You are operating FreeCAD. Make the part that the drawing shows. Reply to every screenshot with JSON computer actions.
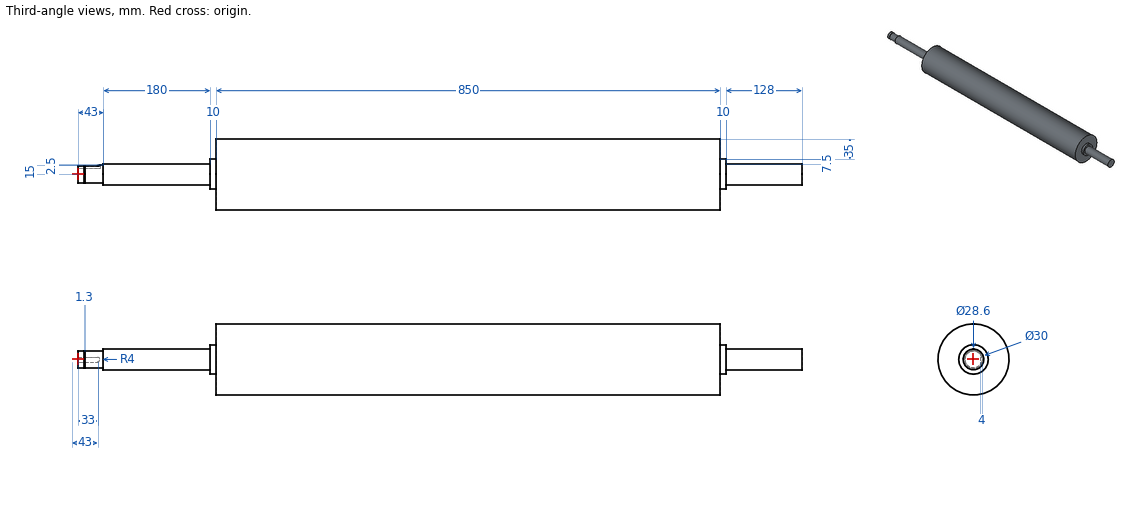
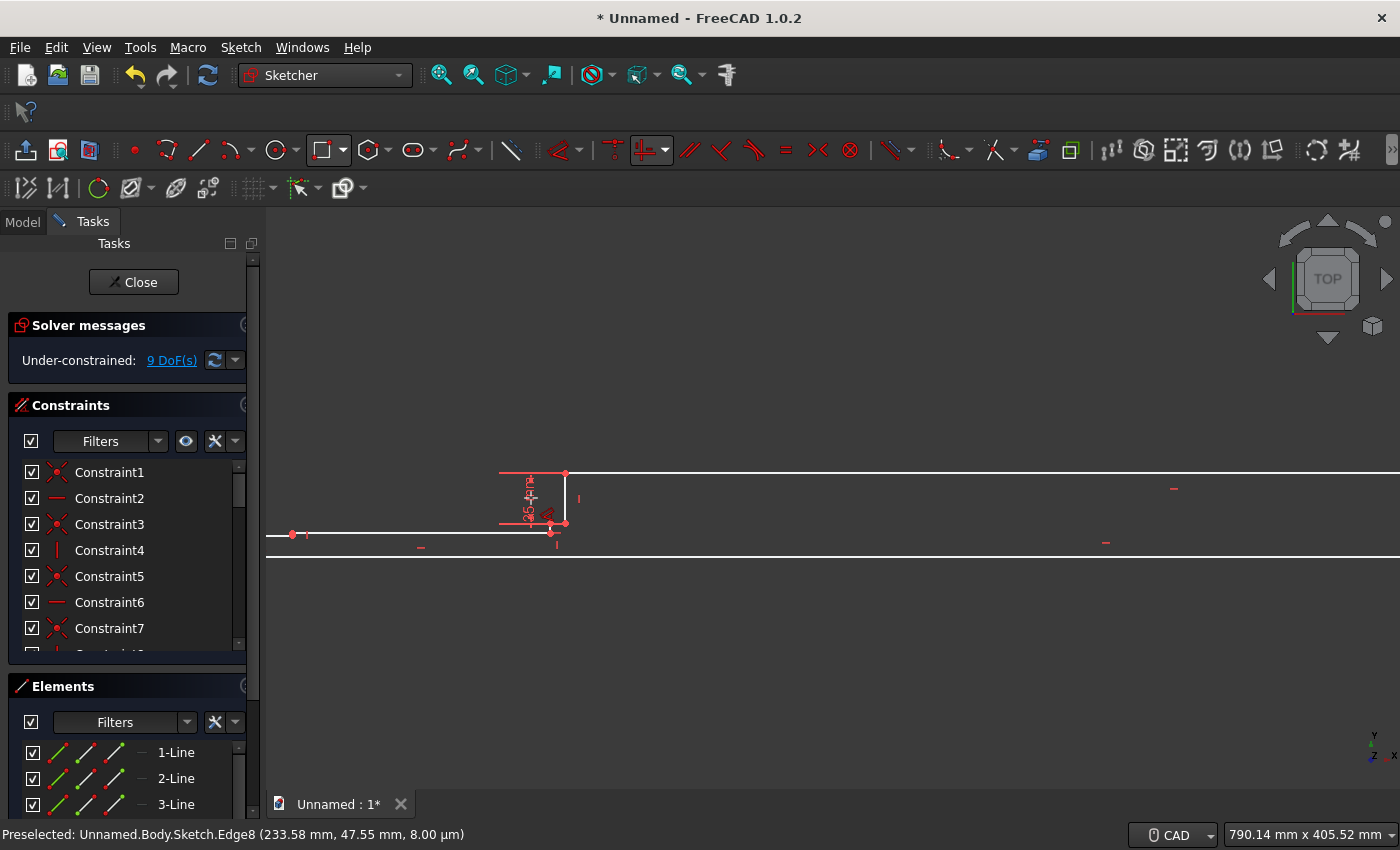
{"action": "scroll", "coordinate": [558, 524], "scroll_direction": "up", "scroll_amount": 6}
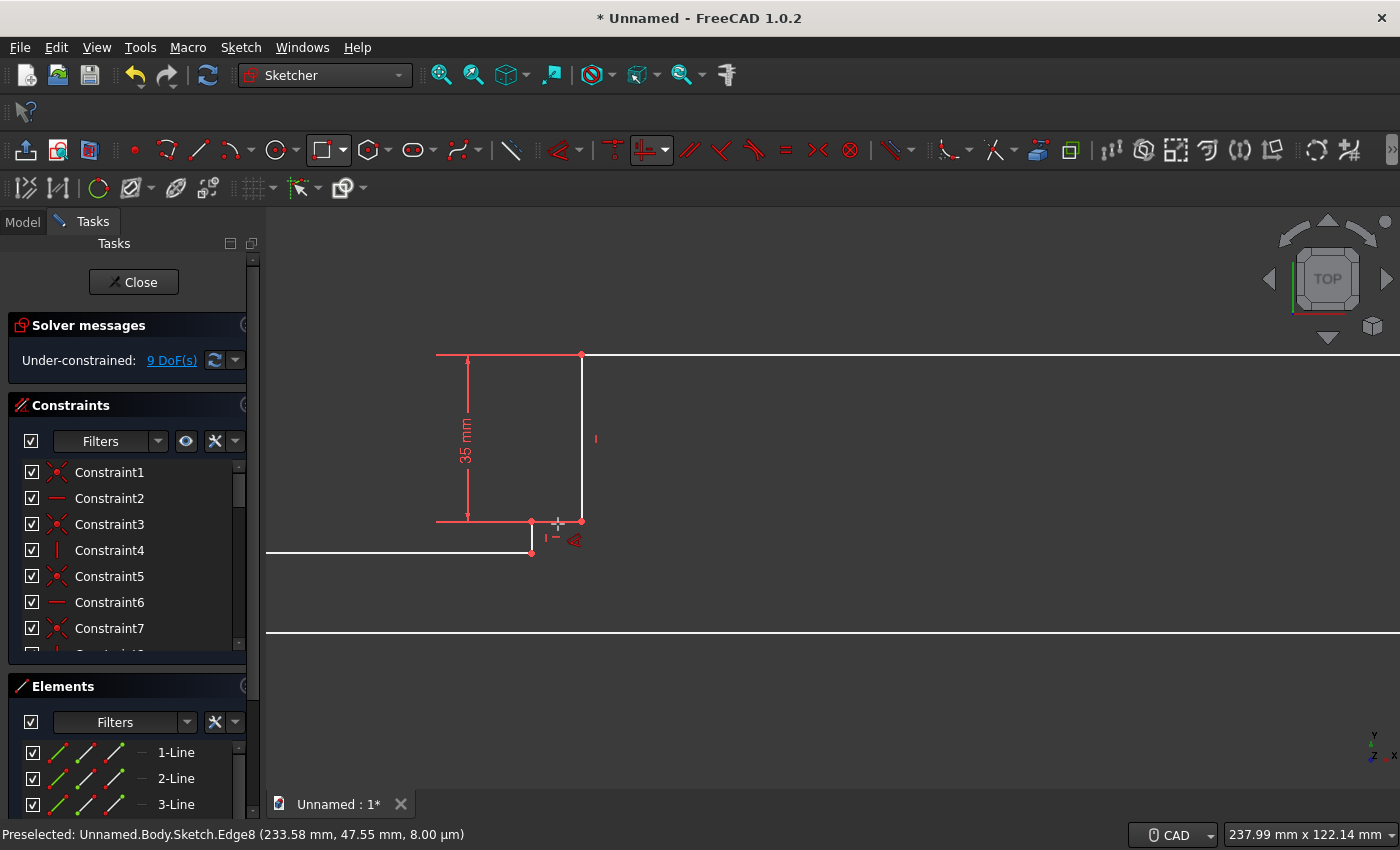
{"action": "left_click", "coordinate": [557, 522]}
{"action": "left_click", "coordinate": [557, 556]}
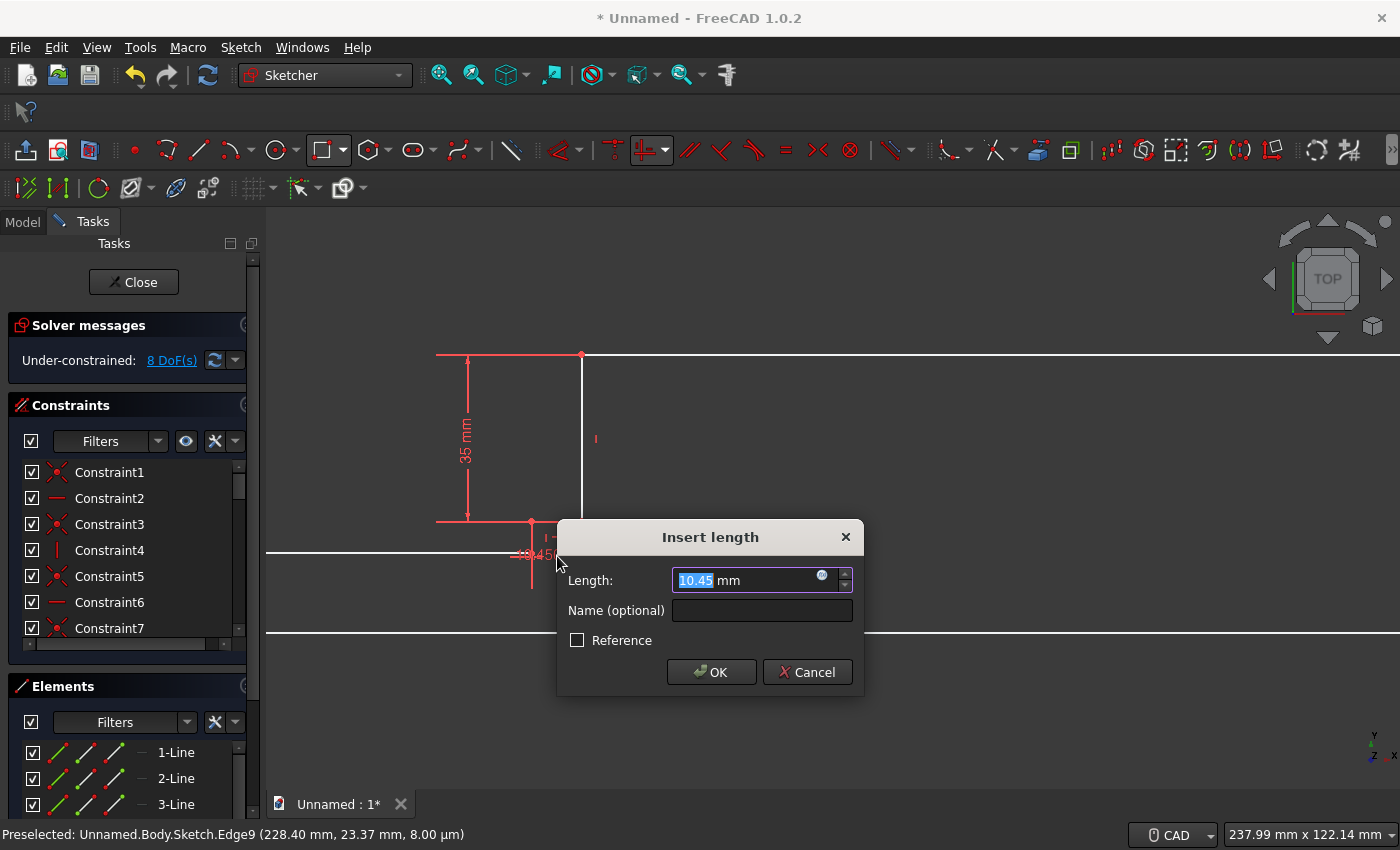
{"action": "type", "text": "10"}
{"action": "key", "text": "Return"}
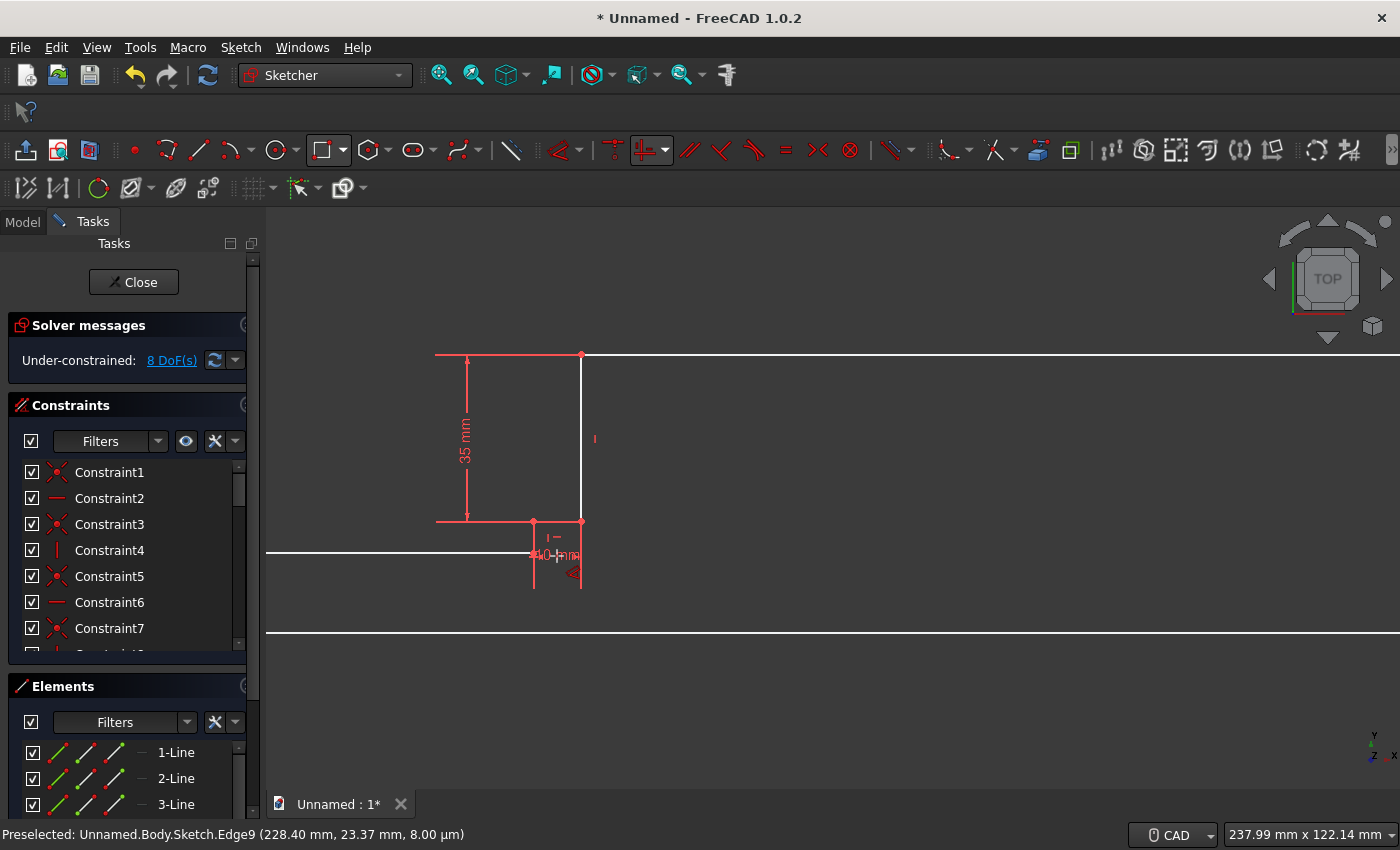
{"action": "scroll", "coordinate": [563, 499], "scroll_direction": "down", "scroll_amount": 11}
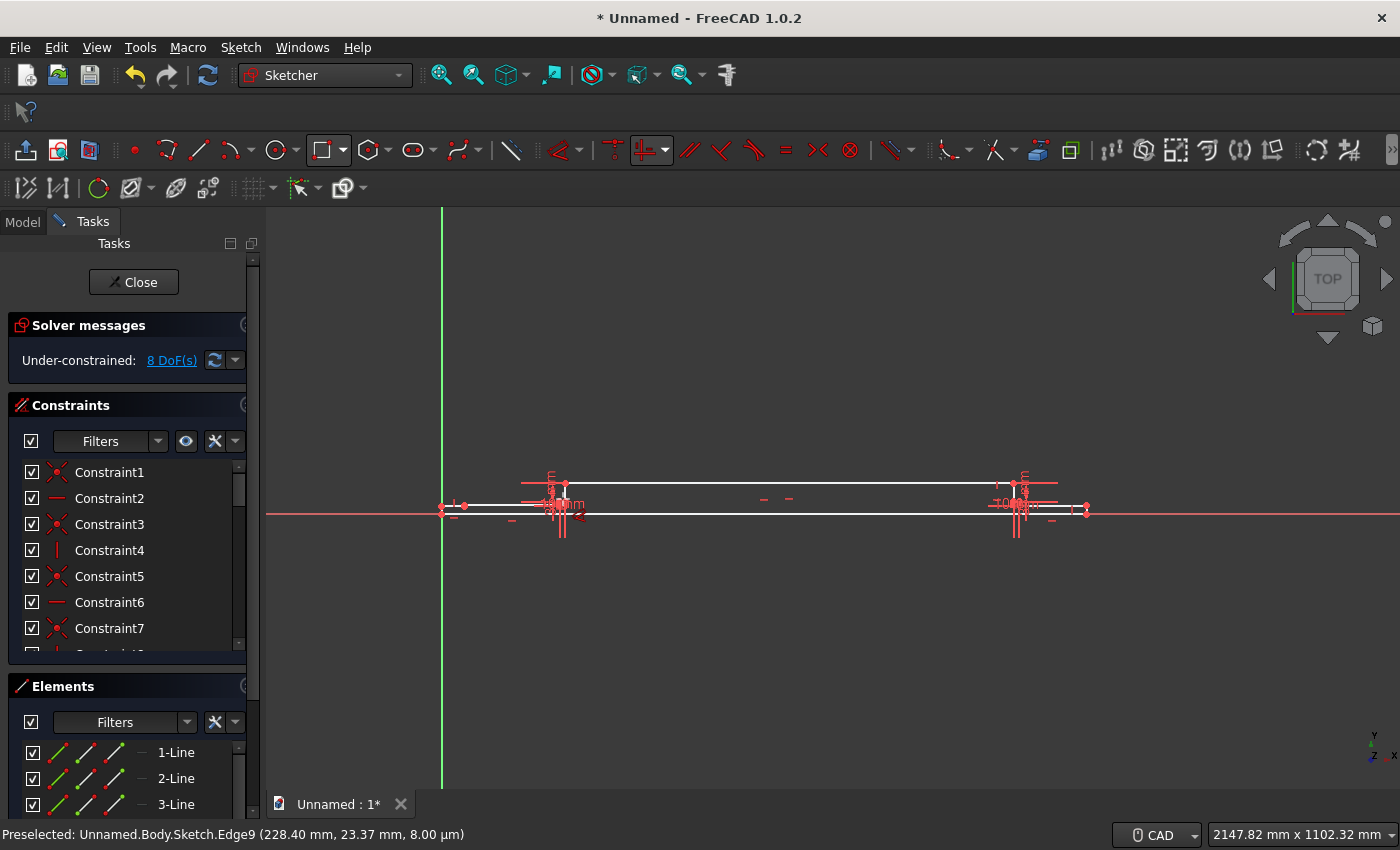
{"action": "scroll", "coordinate": [458, 506], "scroll_direction": "up", "scroll_amount": 4}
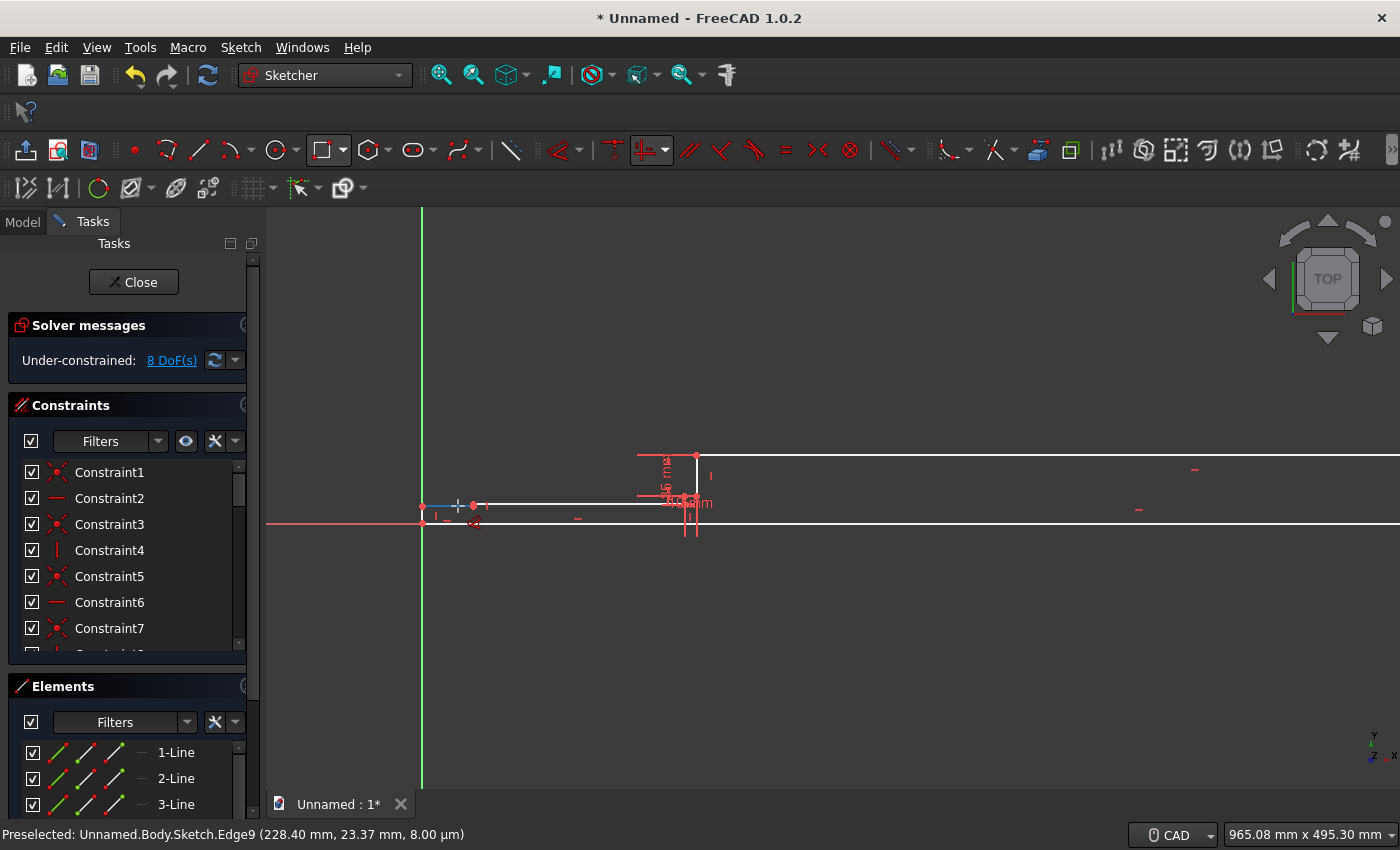
{"action": "left_click", "coordinate": [458, 506]}
{"action": "left_click", "coordinate": [448, 540]}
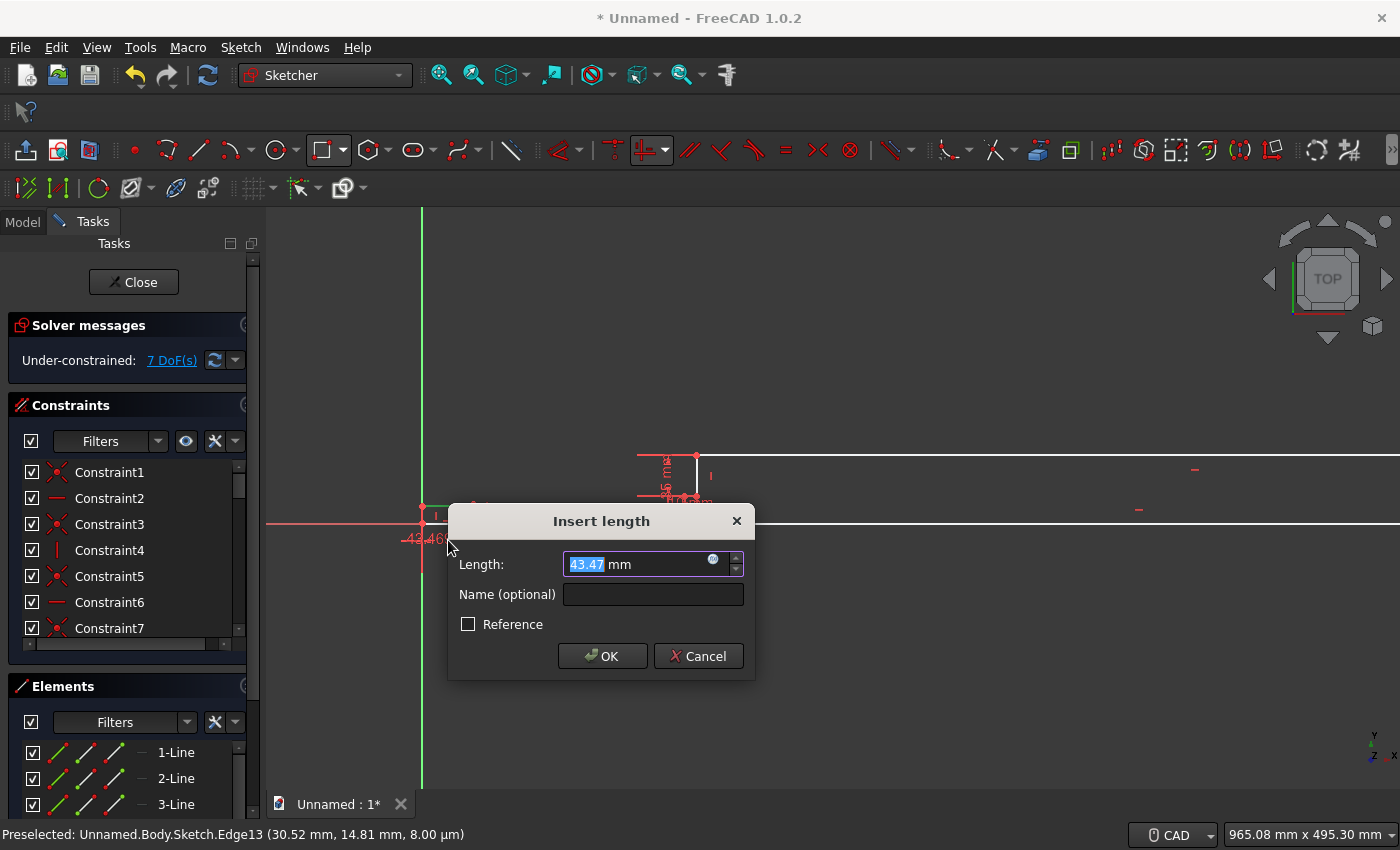
{"action": "type", "text": "43"}
{"action": "key", "text": "Return"}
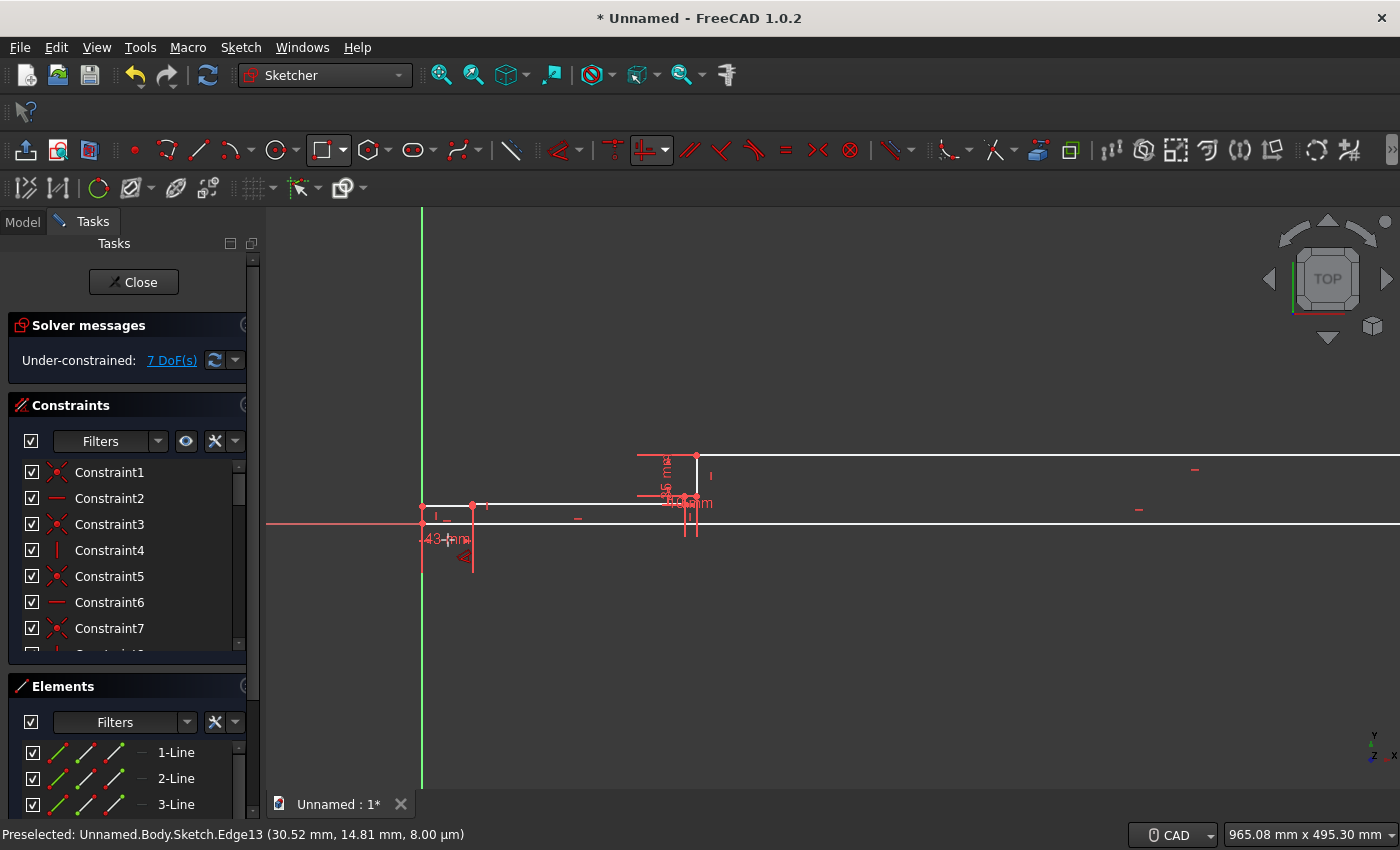
{"action": "scroll", "coordinate": [422, 515], "scroll_direction": "up", "scroll_amount": 5}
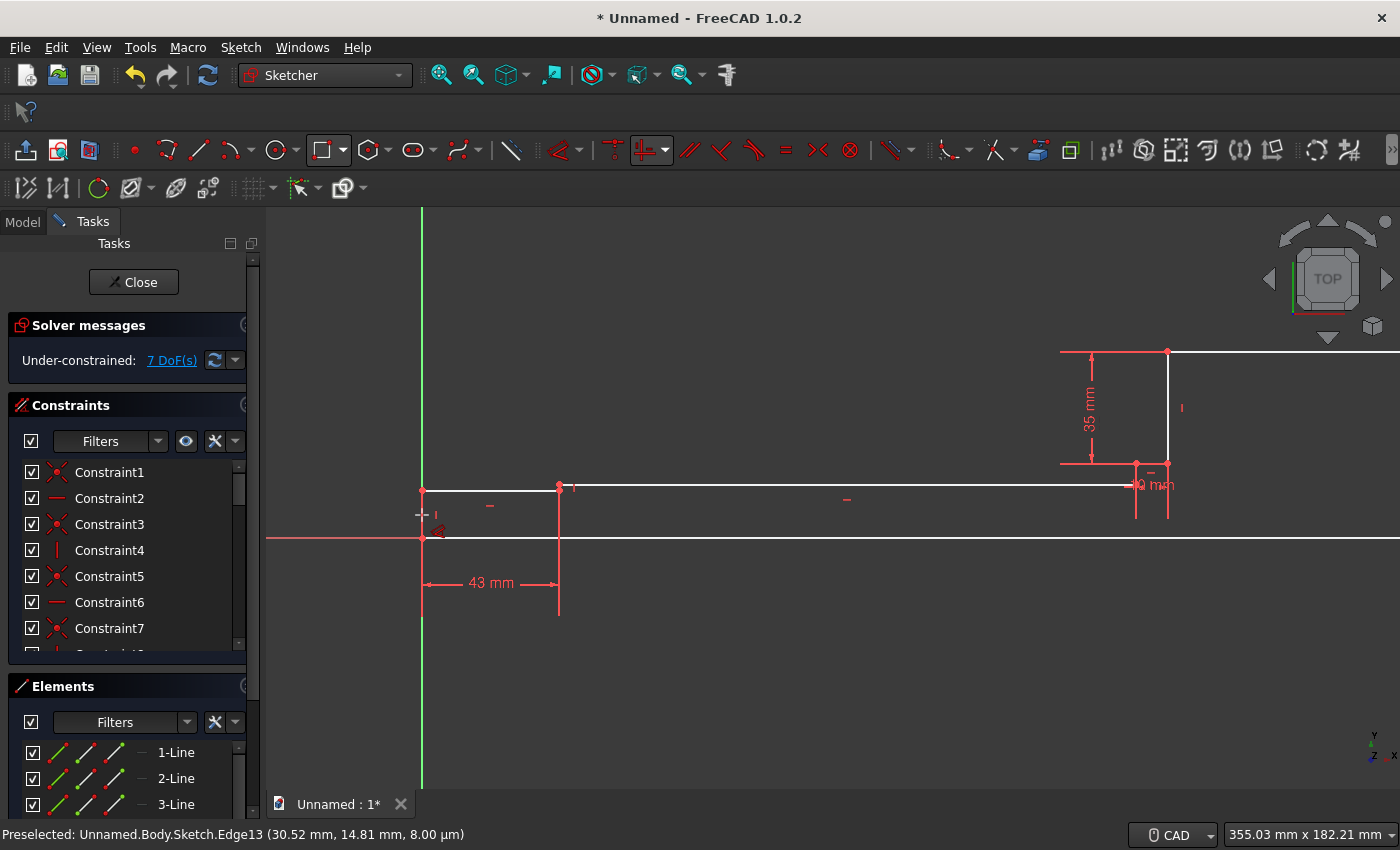
{"action": "left_click", "coordinate": [422, 514]}
{"action": "left_click", "coordinate": [388, 514]}